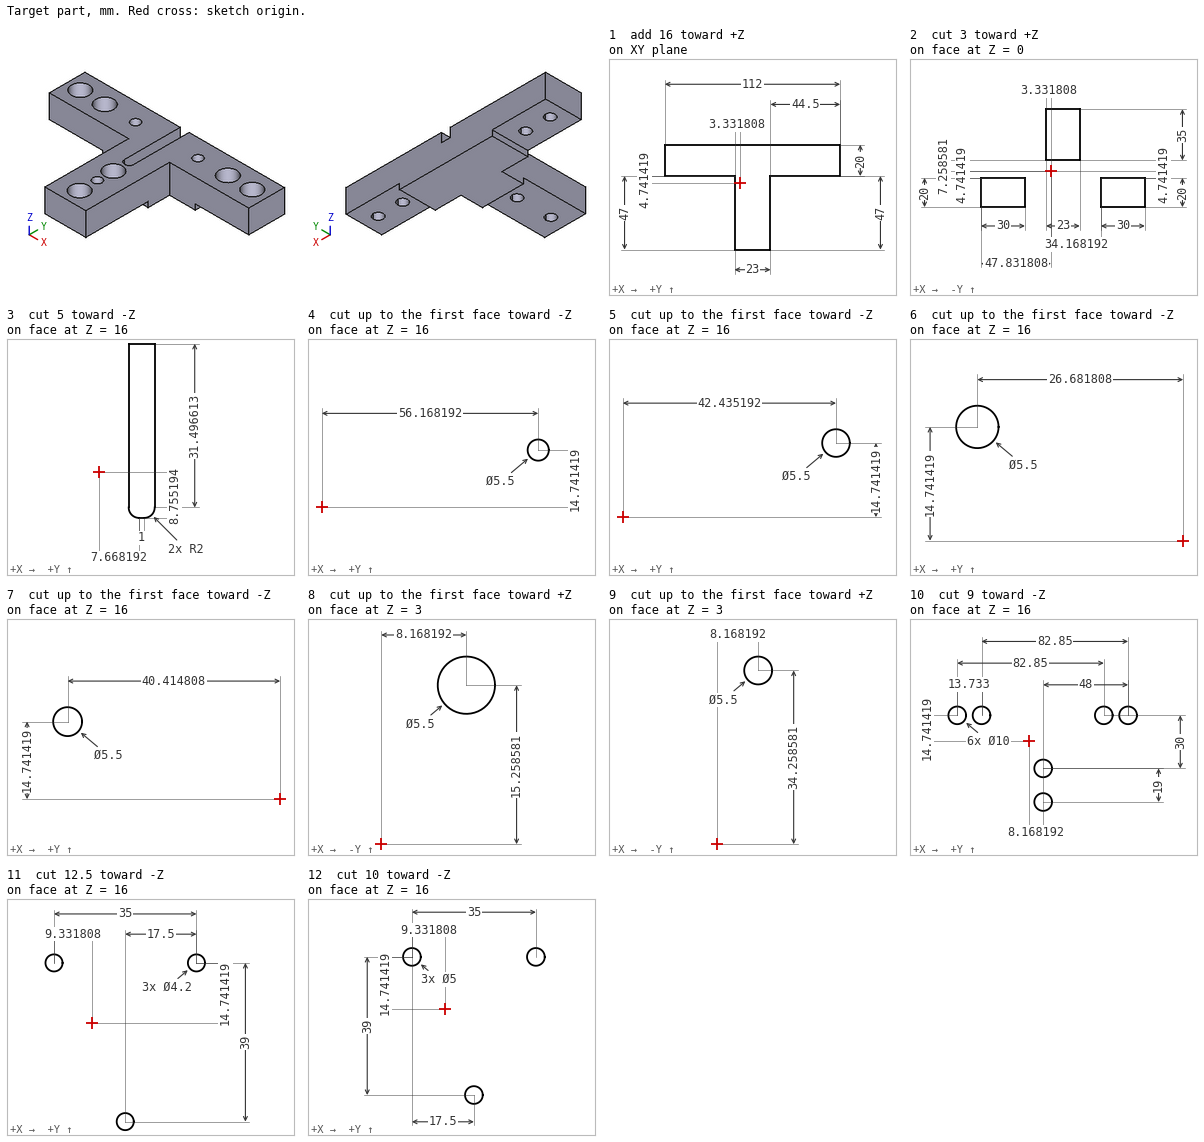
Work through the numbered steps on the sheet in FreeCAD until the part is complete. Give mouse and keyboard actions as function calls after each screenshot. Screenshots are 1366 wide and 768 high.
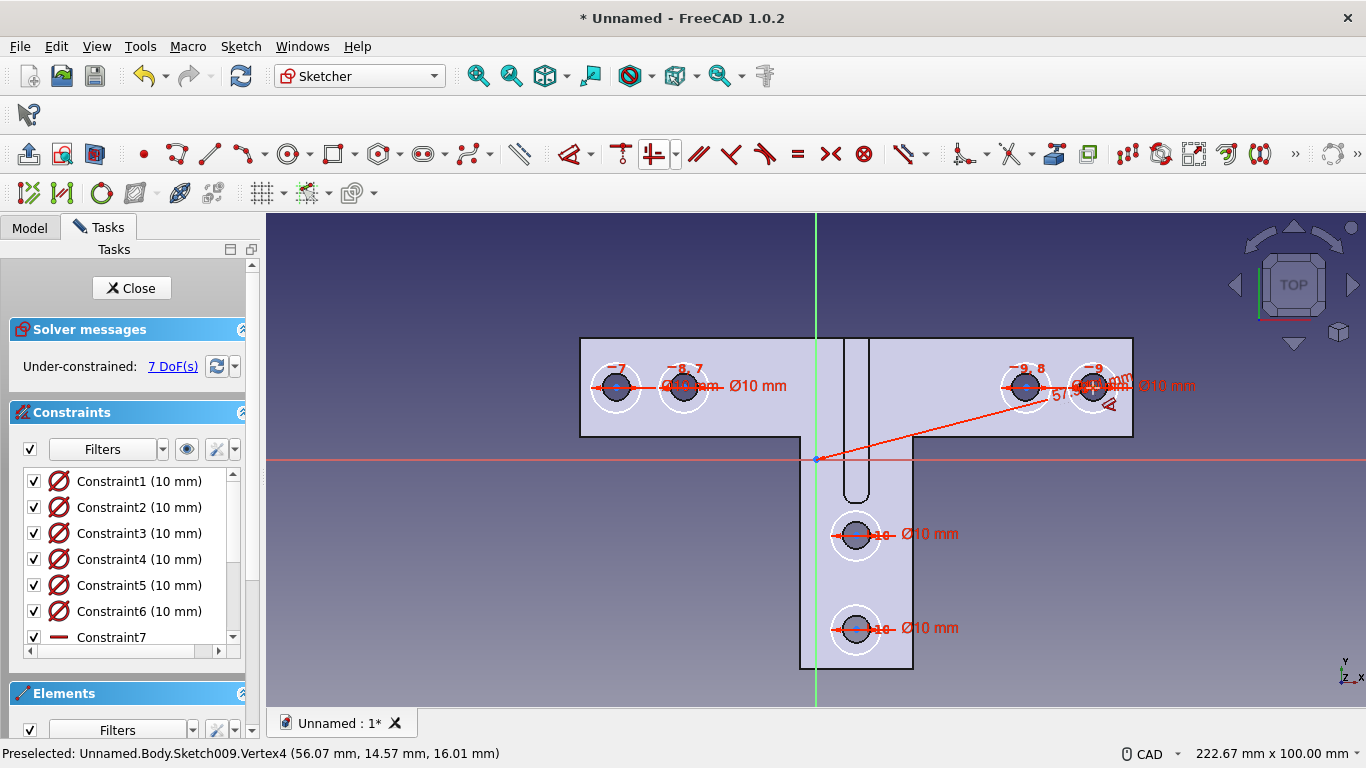
click(856, 536)
click(975, 354)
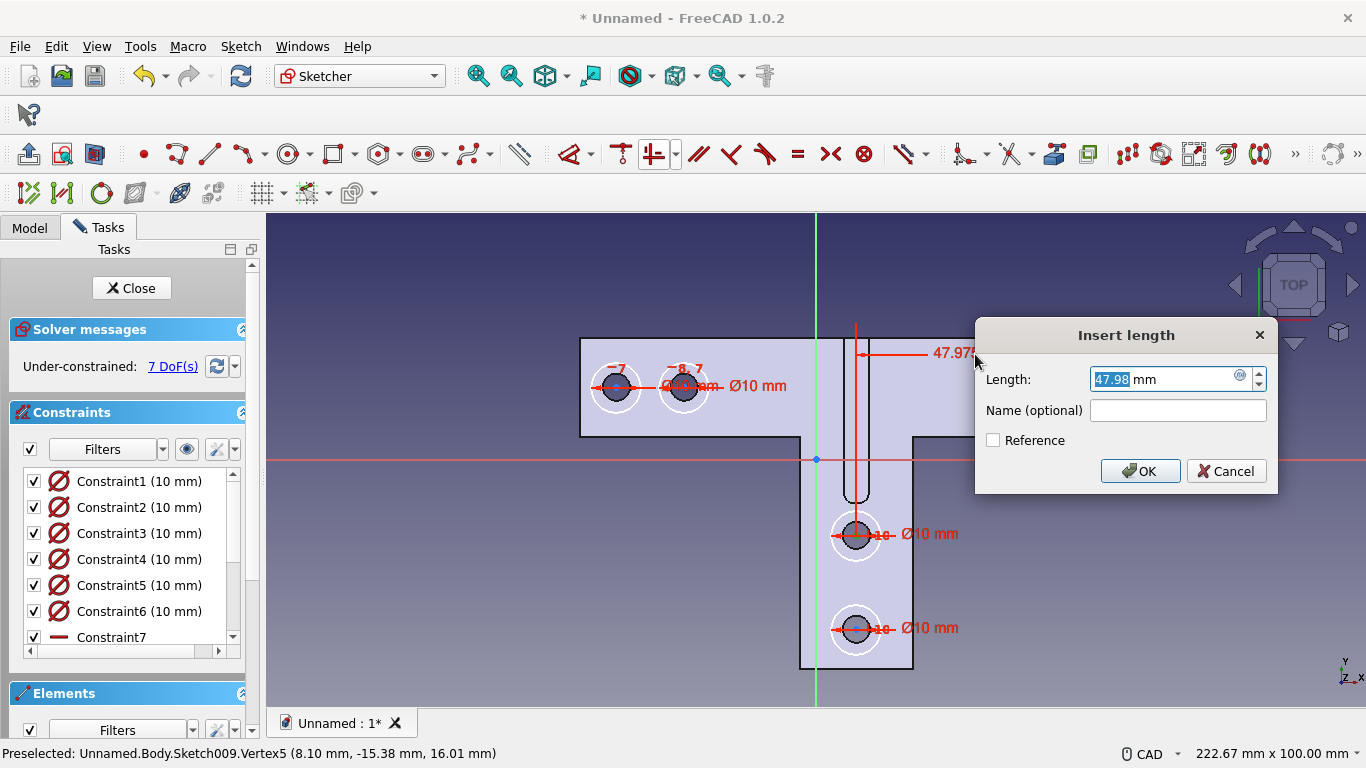
text(48)
key(Return)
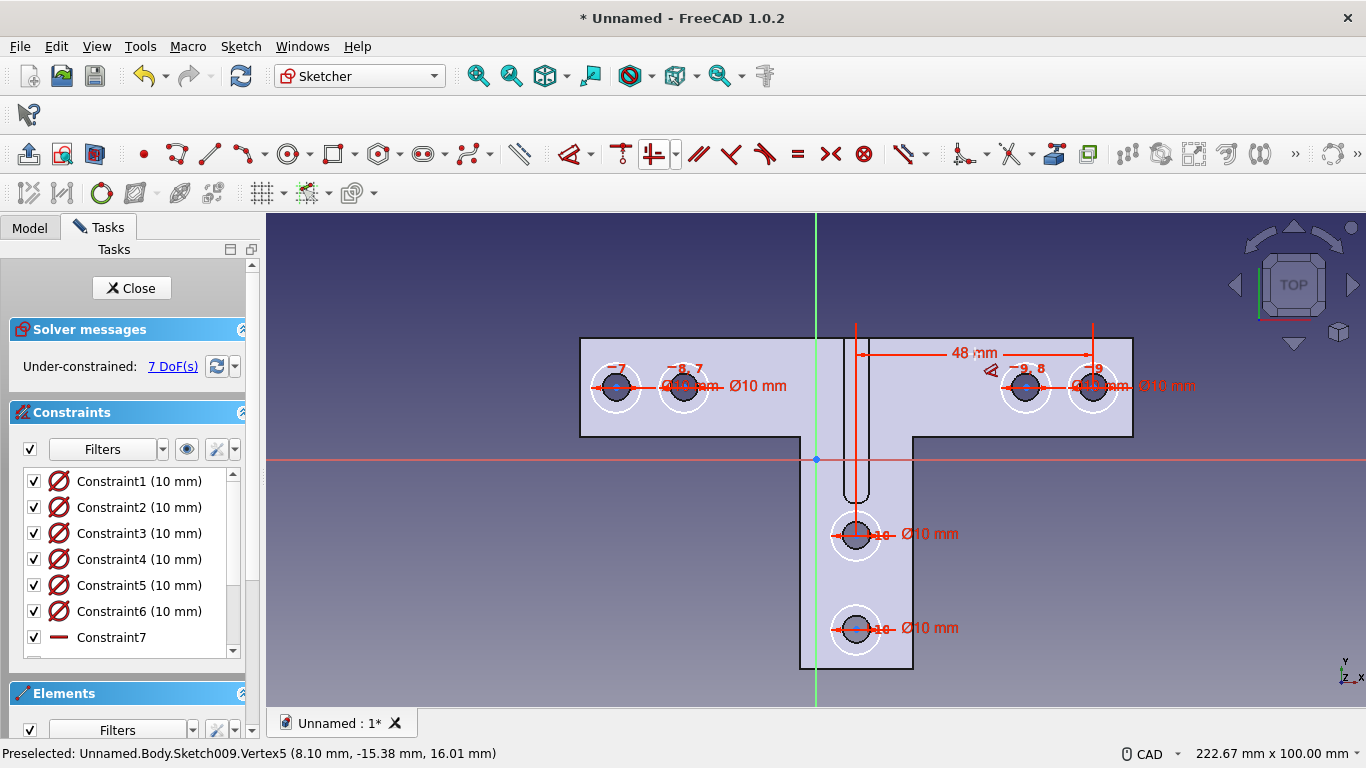
click(1026, 388)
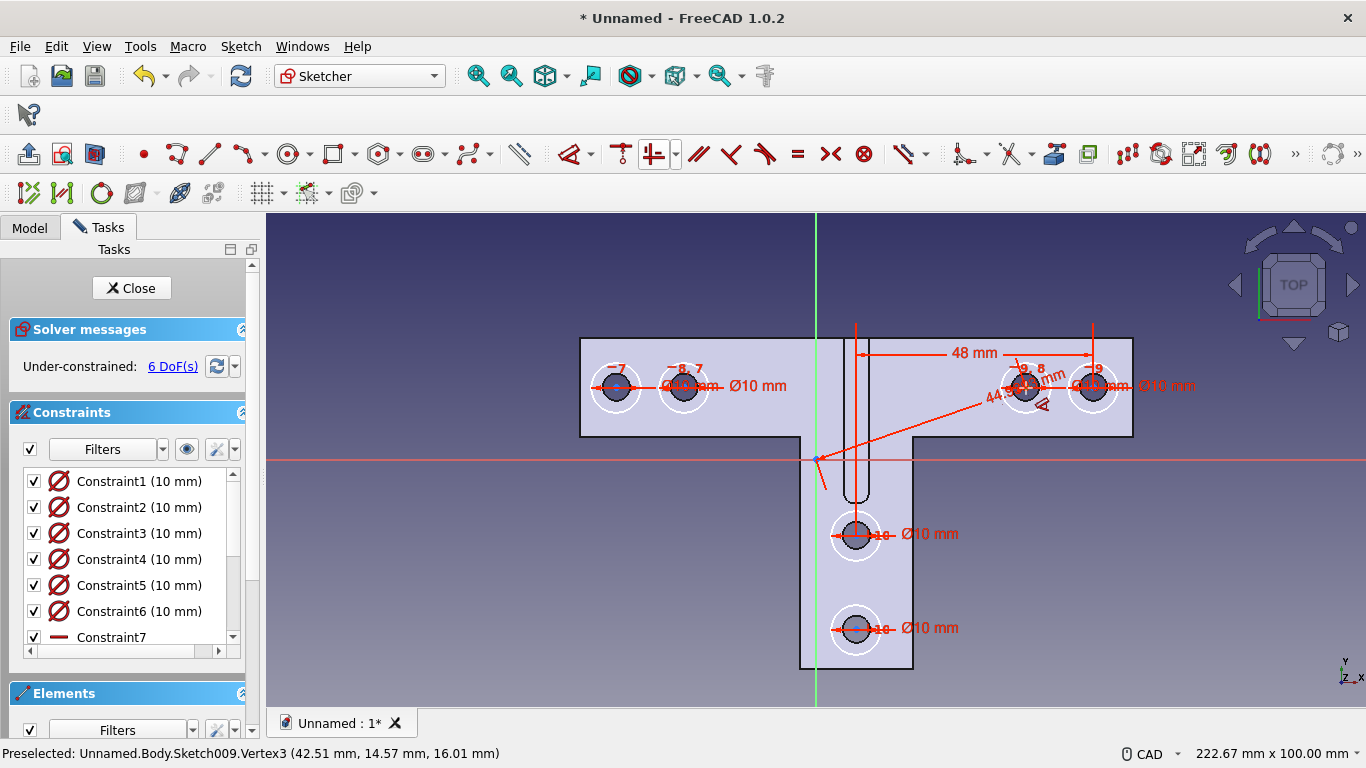
click(856, 536)
click(1060, 428)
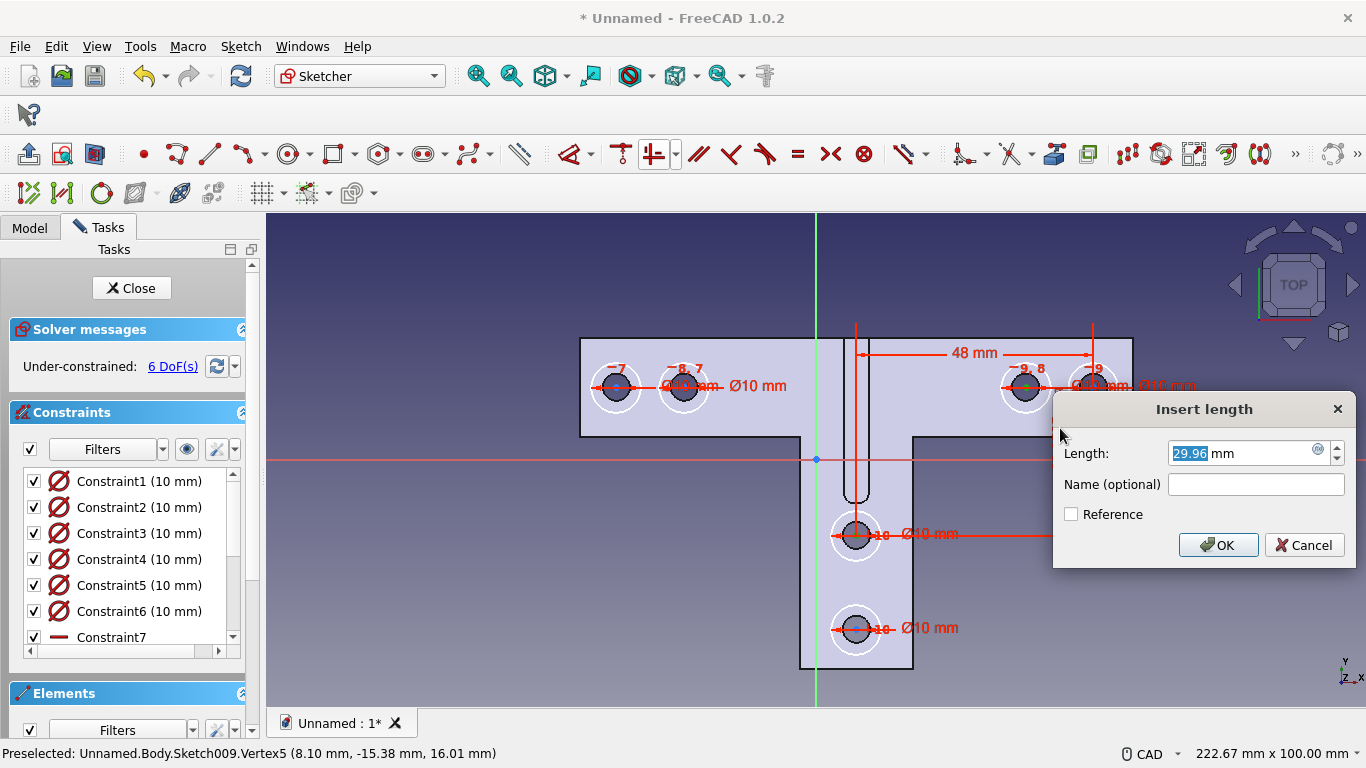
text(30)
key(Return)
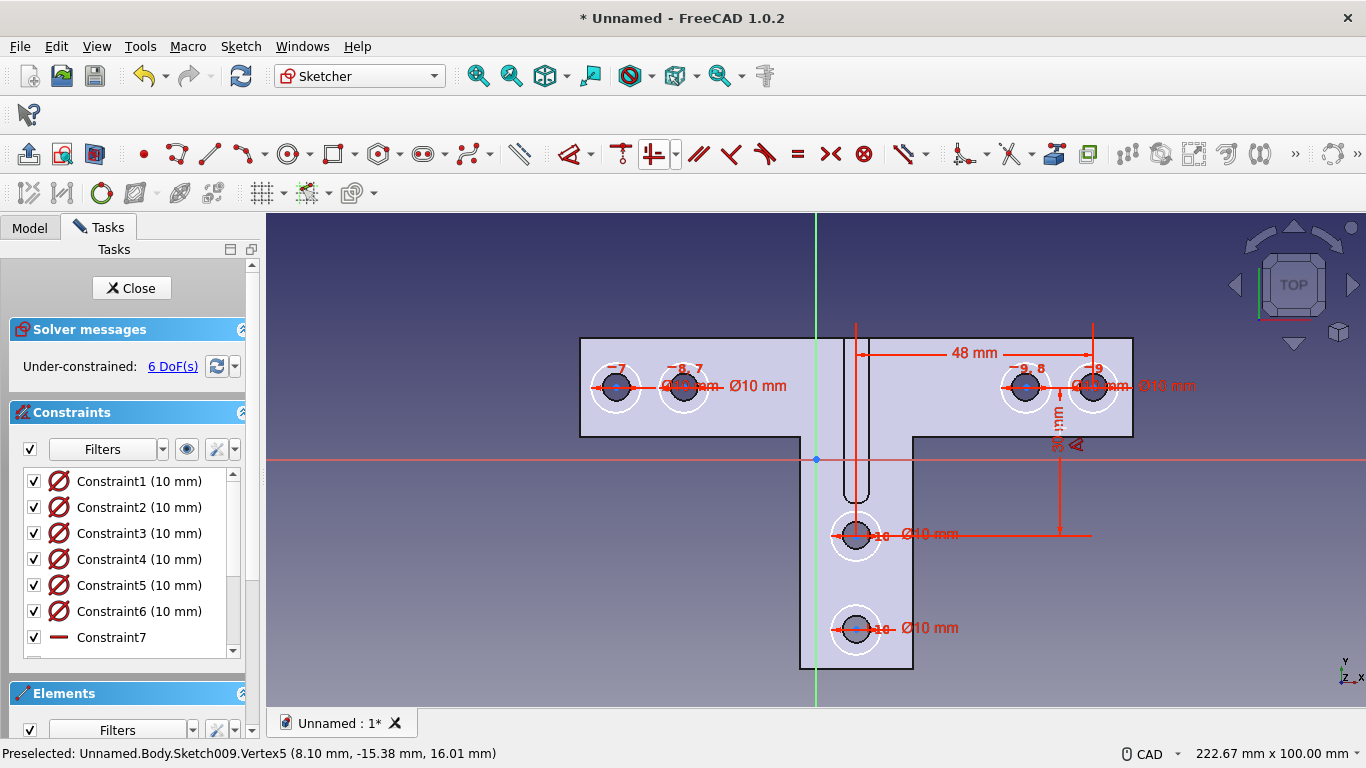
click(856, 536)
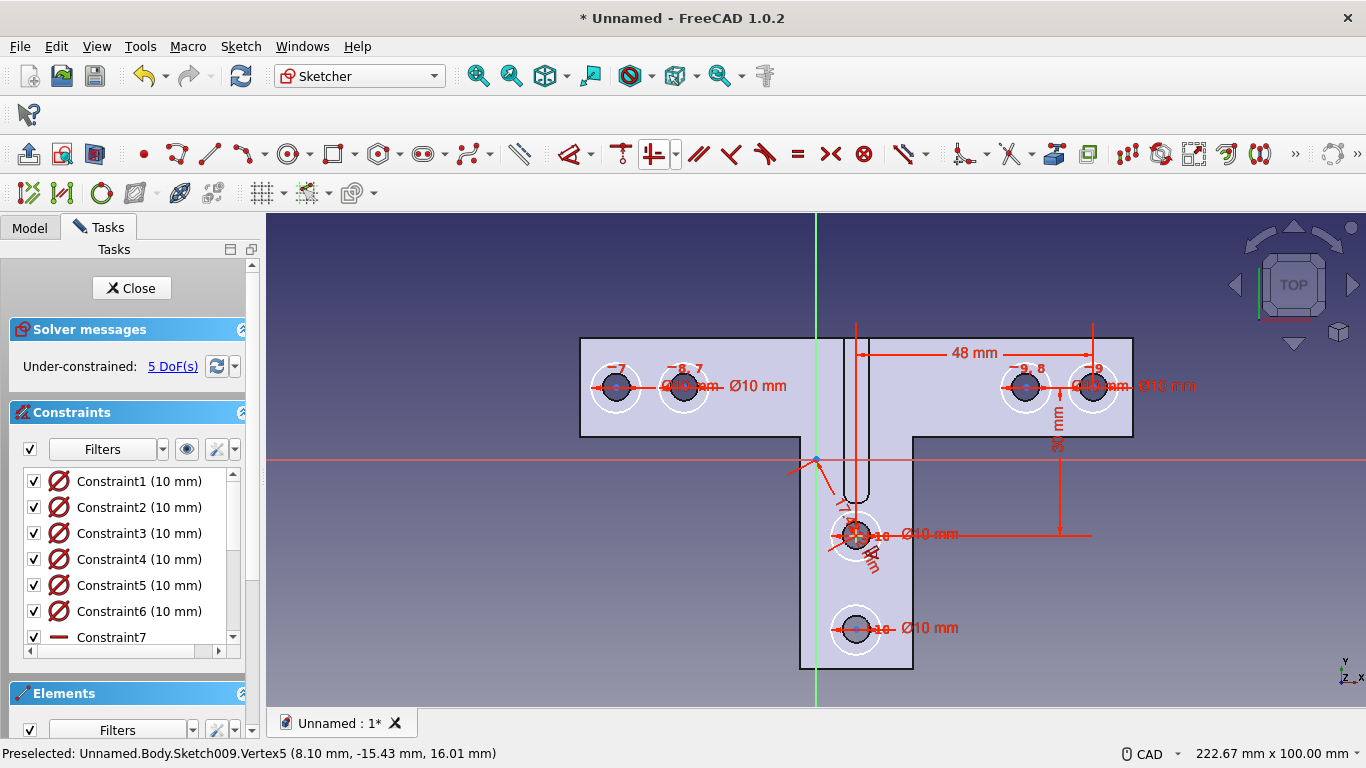
click(856, 630)
click(890, 583)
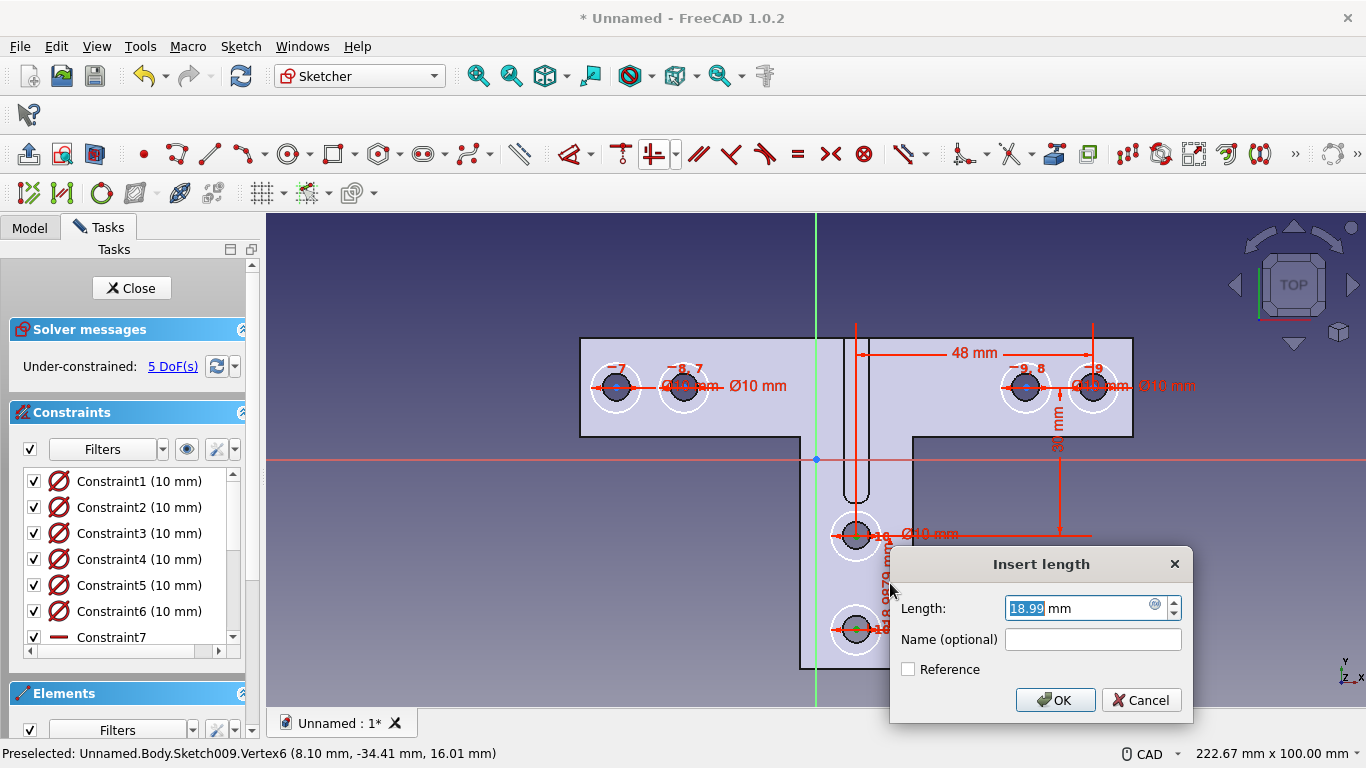
text(19)
key(Return)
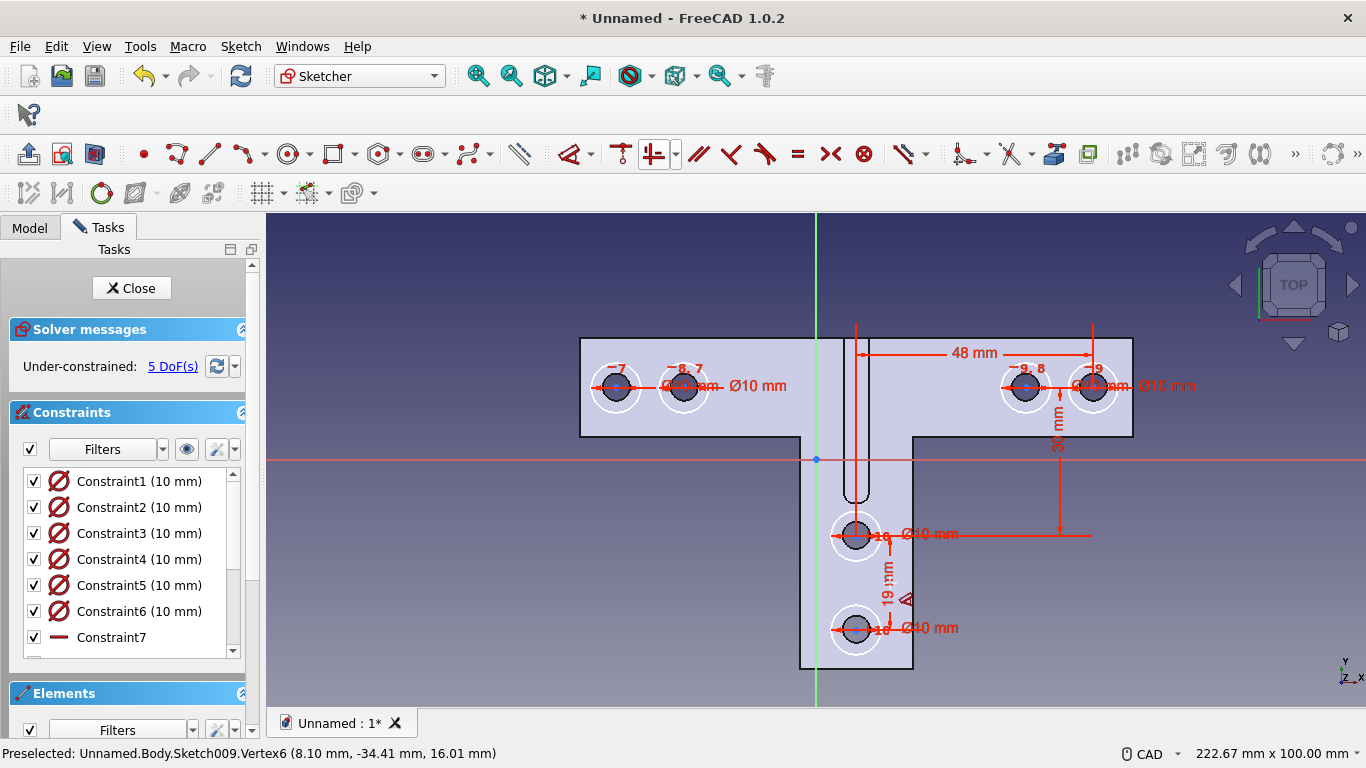
click(616, 388)